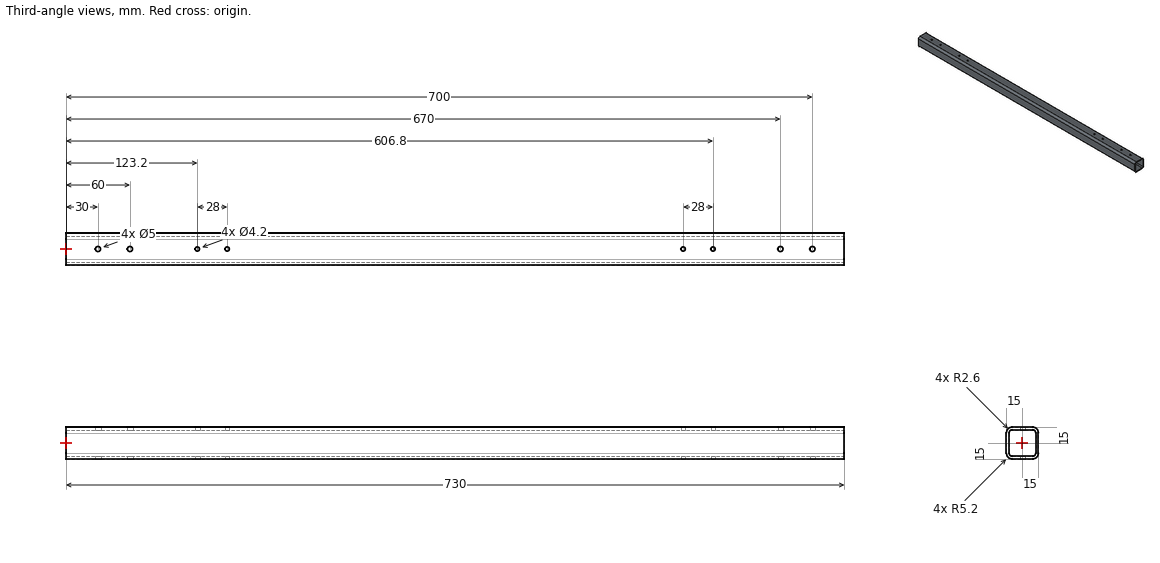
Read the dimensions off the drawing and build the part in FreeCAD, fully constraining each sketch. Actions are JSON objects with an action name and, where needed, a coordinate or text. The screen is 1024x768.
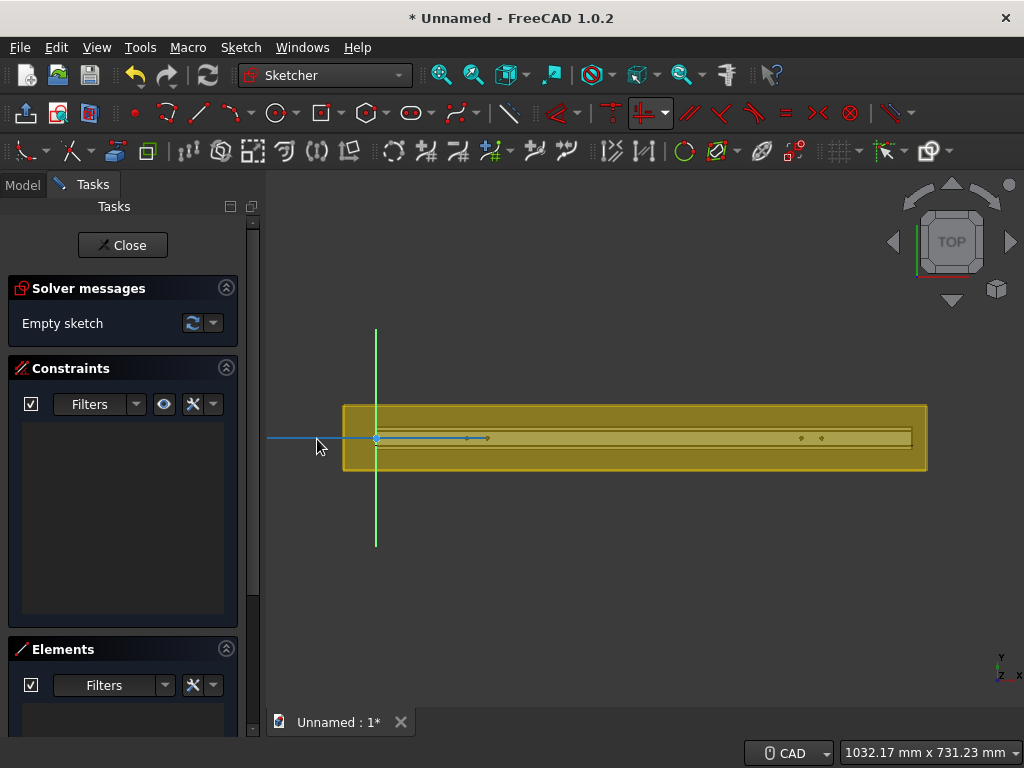
{"action": "left_click", "coordinate": [276, 114]}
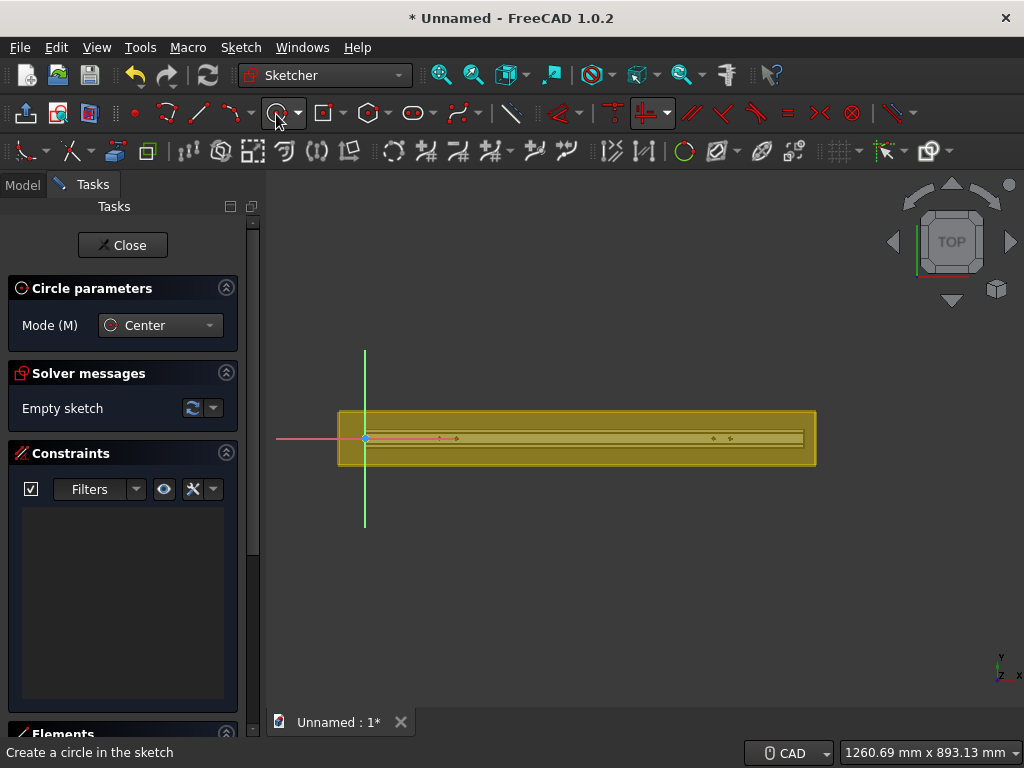
{"action": "scroll", "coordinate": [383, 439], "scroll_direction": "up", "scroll_amount": 14}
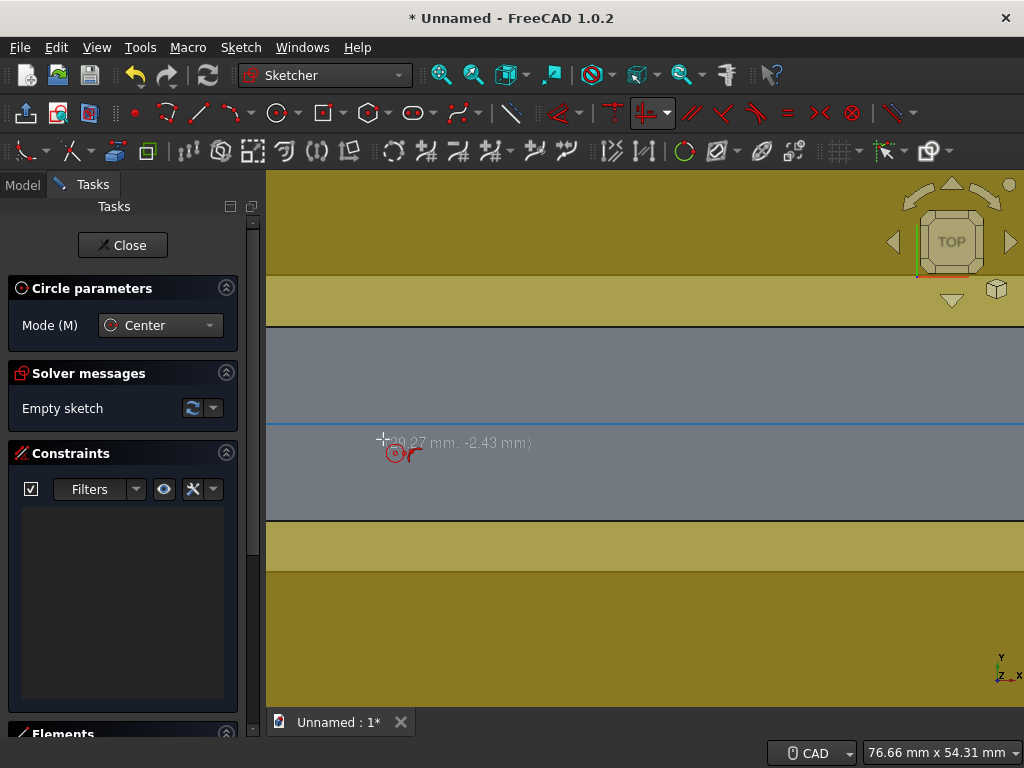
{"action": "scroll", "coordinate": [383, 439], "scroll_direction": "down", "scroll_amount": 14}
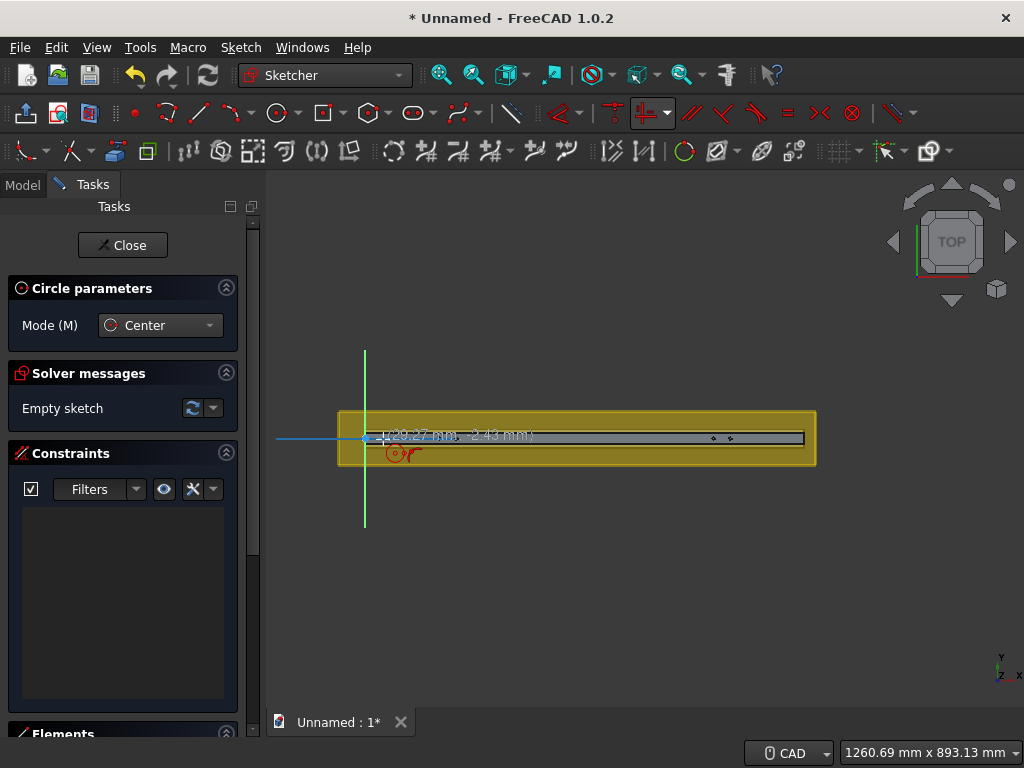
{"action": "left_click", "coordinate": [383, 439]}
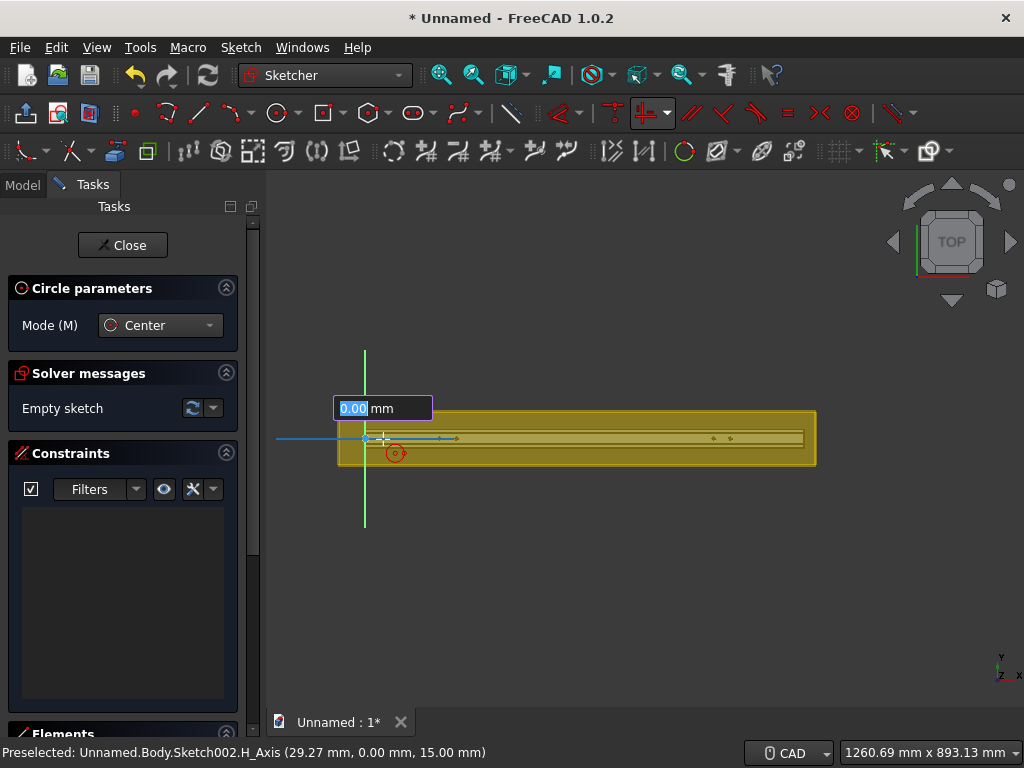
{"action": "scroll", "coordinate": [383, 440], "scroll_direction": "up", "scroll_amount": 13}
{"action": "mouse_move", "coordinate": [380, 433]}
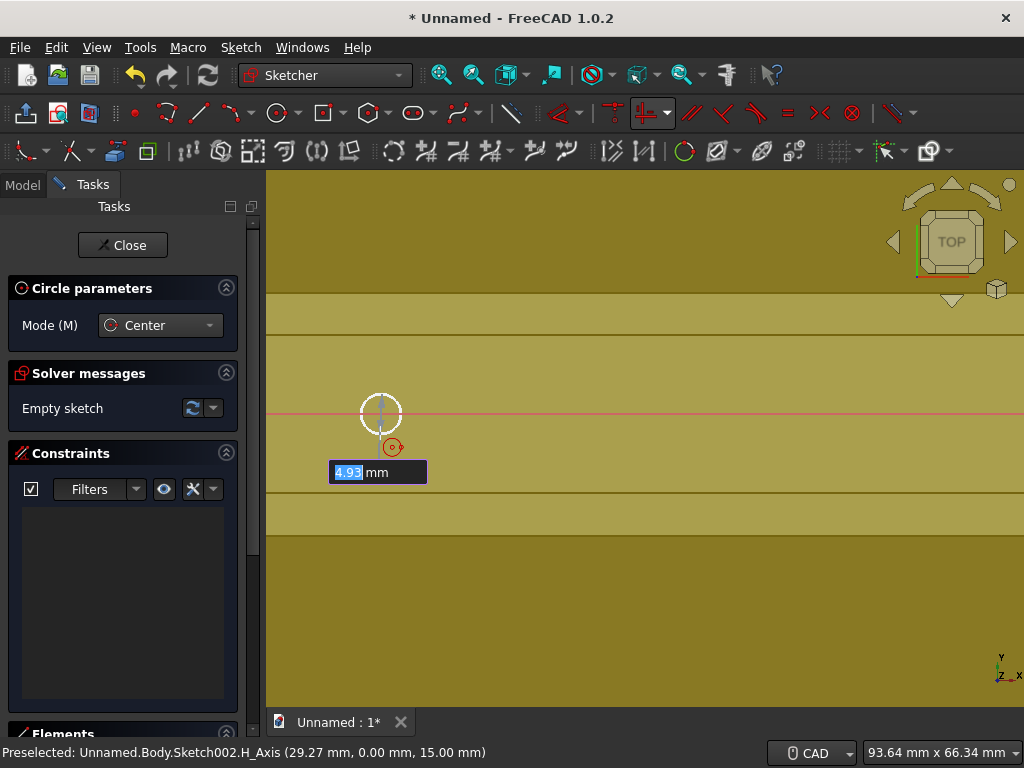
{"action": "type", "text": "5"}
{"action": "key", "text": "Return"}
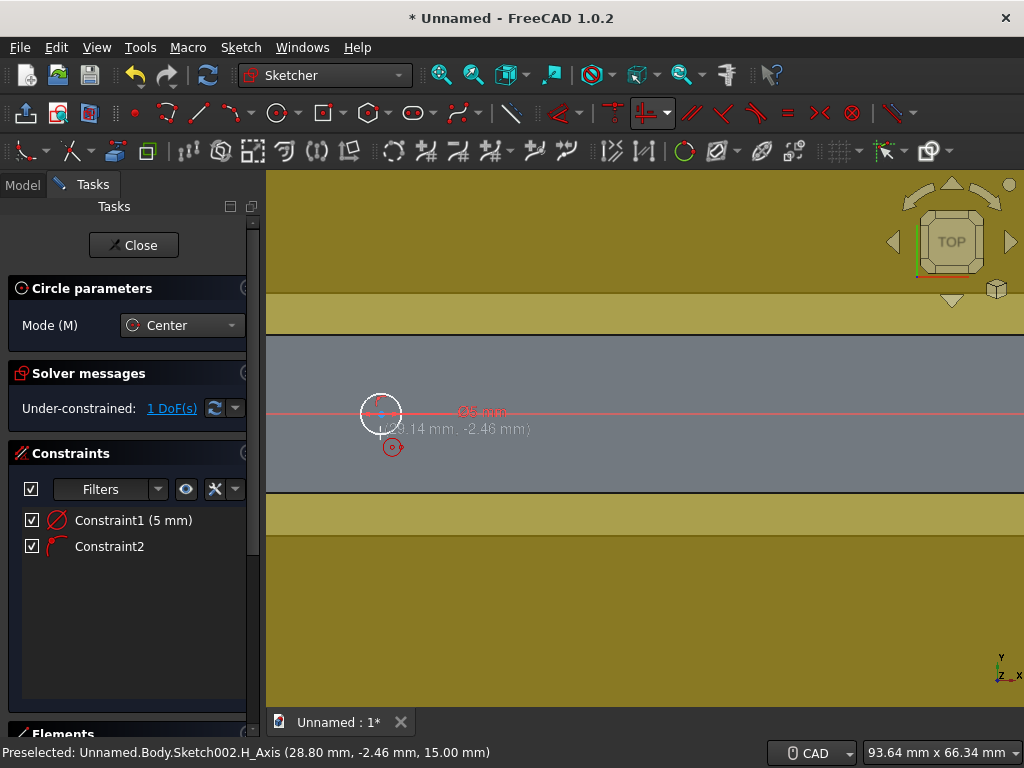
{"action": "scroll", "coordinate": [383, 440], "scroll_direction": "down", "scroll_amount": 13}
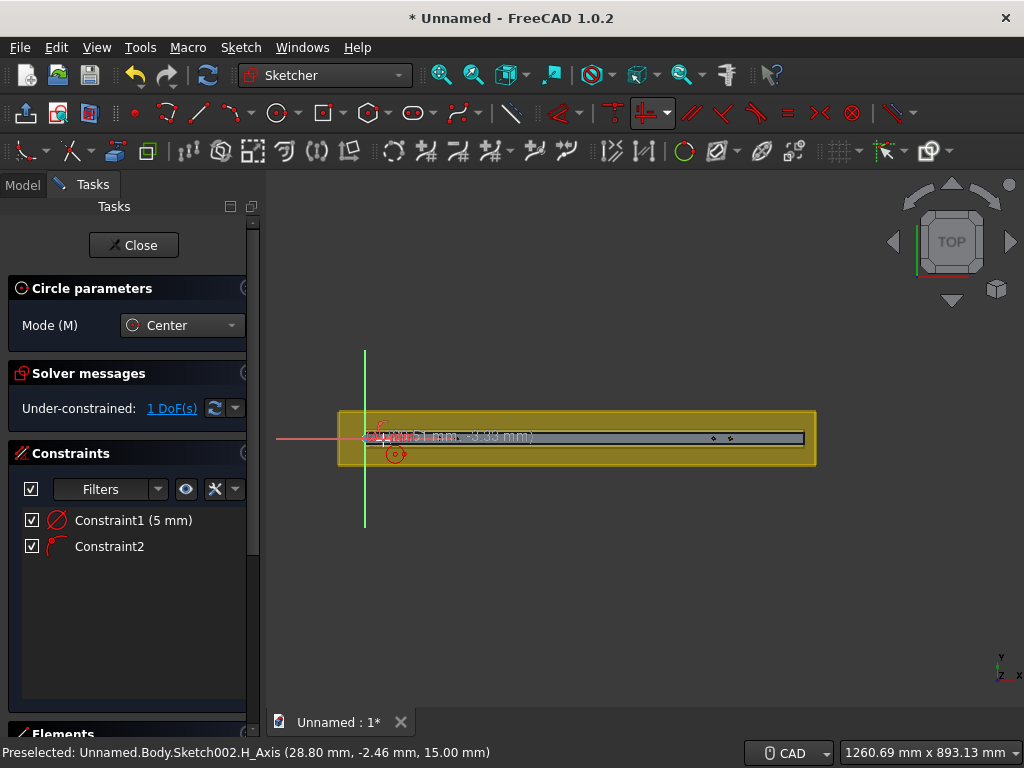
{"action": "left_click", "coordinate": [401, 439]}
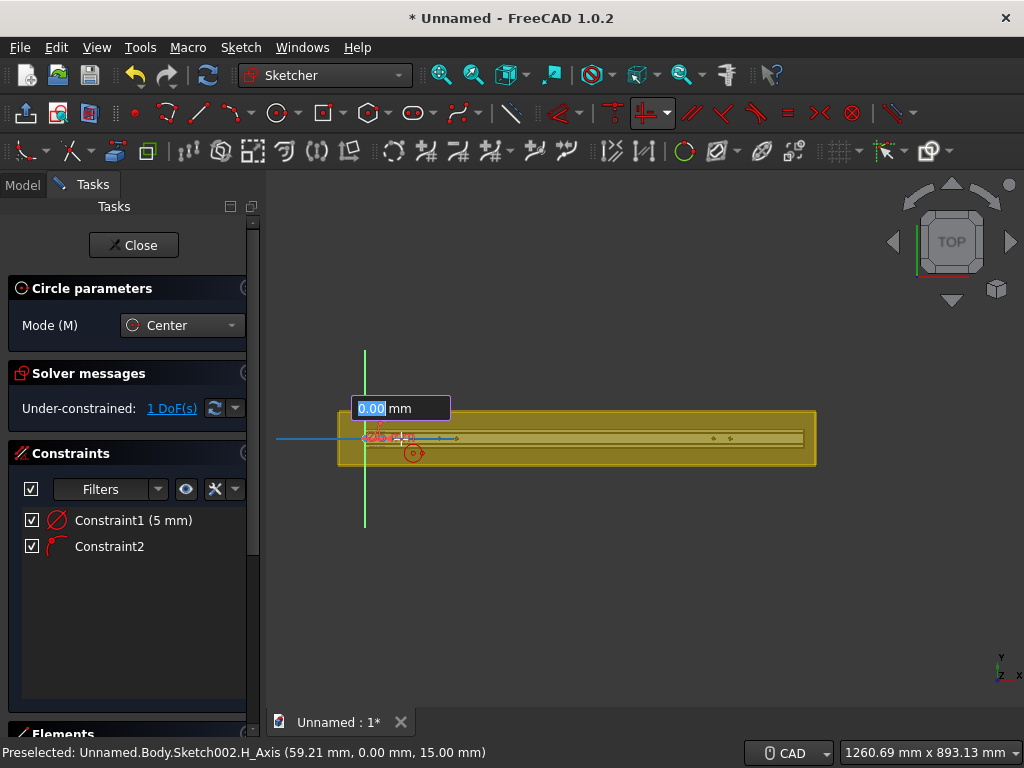
{"action": "scroll", "coordinate": [401, 440], "scroll_direction": "up", "scroll_amount": 13}
{"action": "mouse_move", "coordinate": [398, 433]}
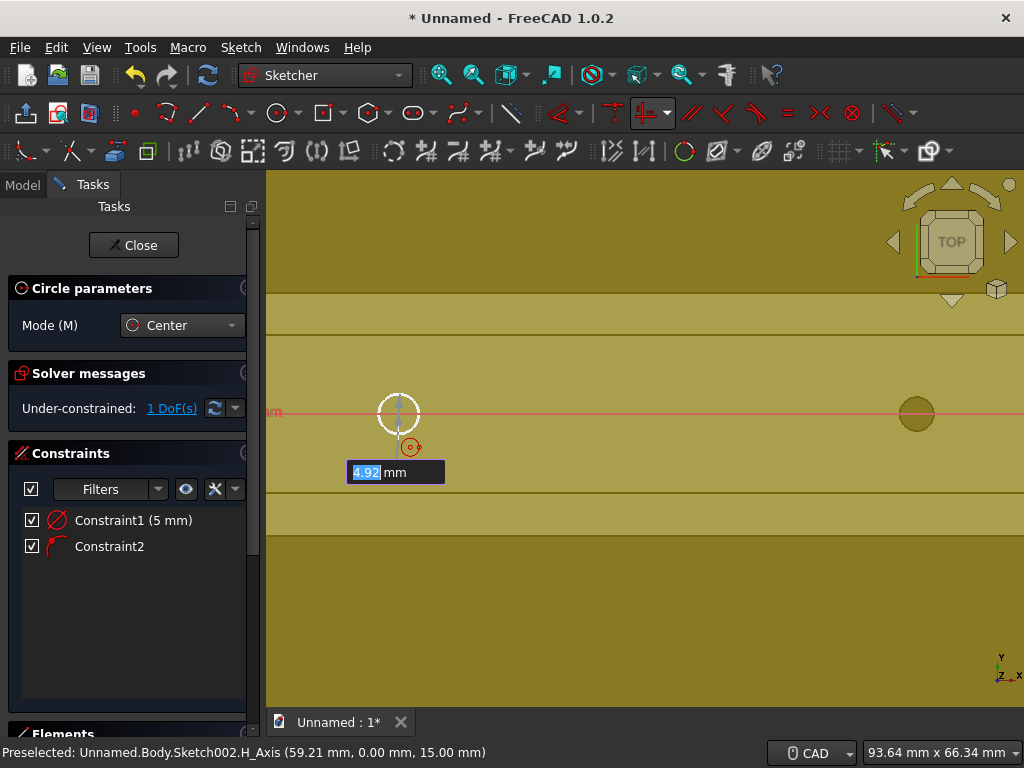
{"action": "type", "text": "5"}
{"action": "key", "text": "Return"}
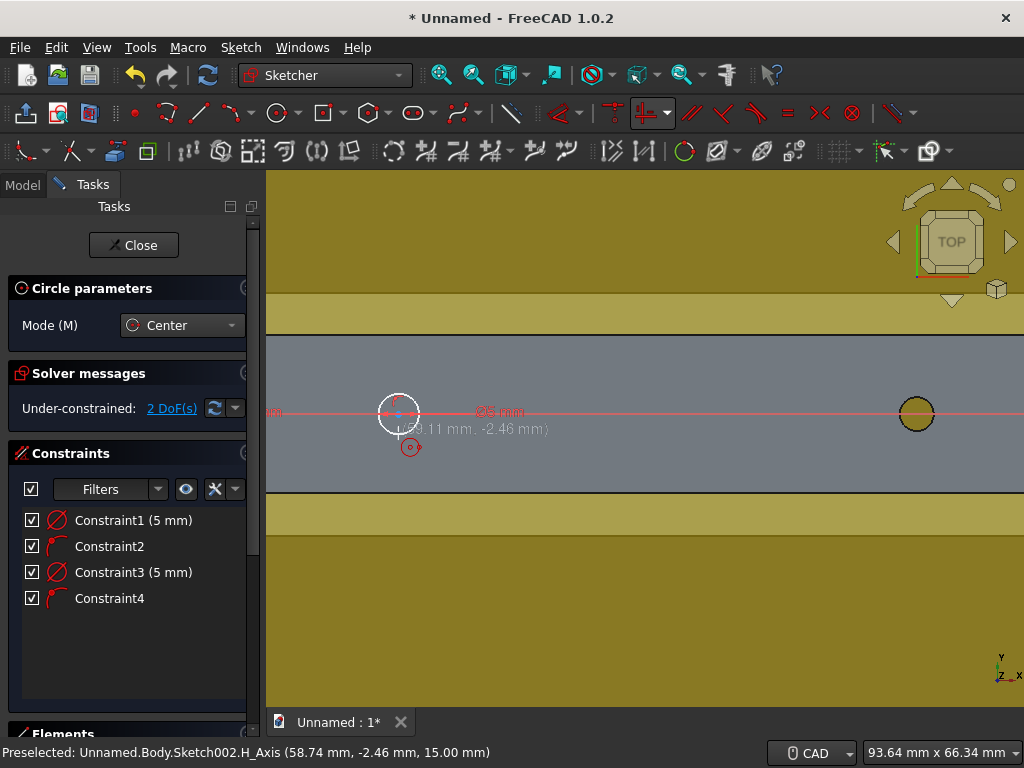
{"action": "scroll", "coordinate": [401, 440], "scroll_direction": "down", "scroll_amount": 13}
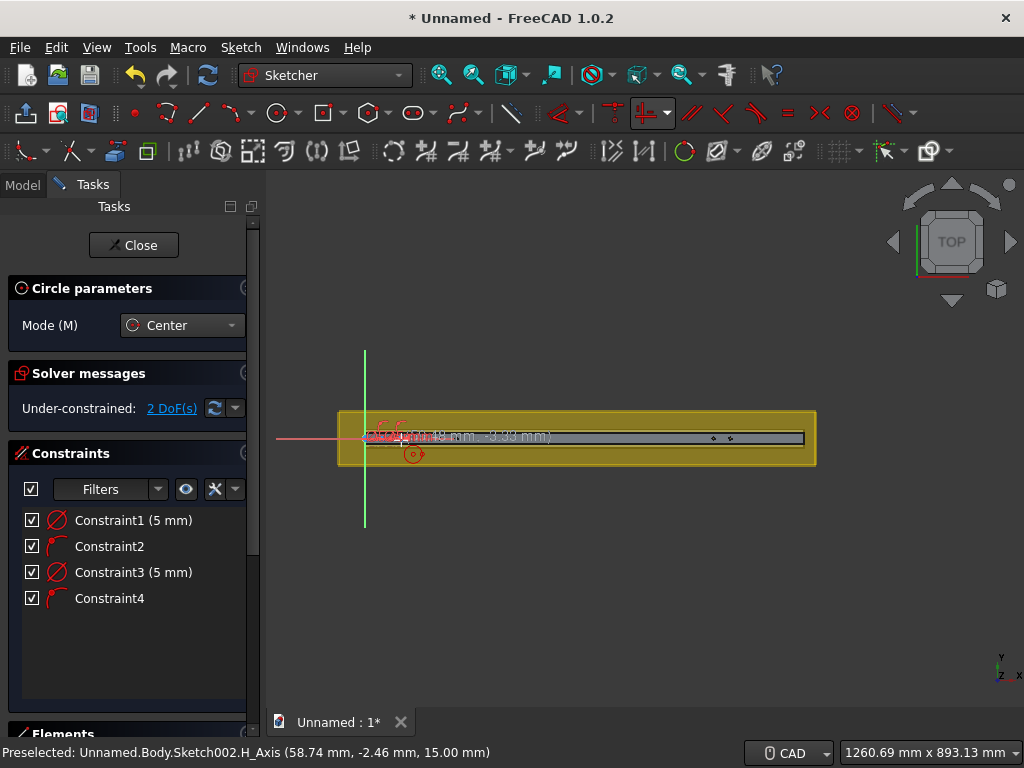
{"action": "scroll", "coordinate": [786, 439], "scroll_direction": "up", "scroll_amount": 14}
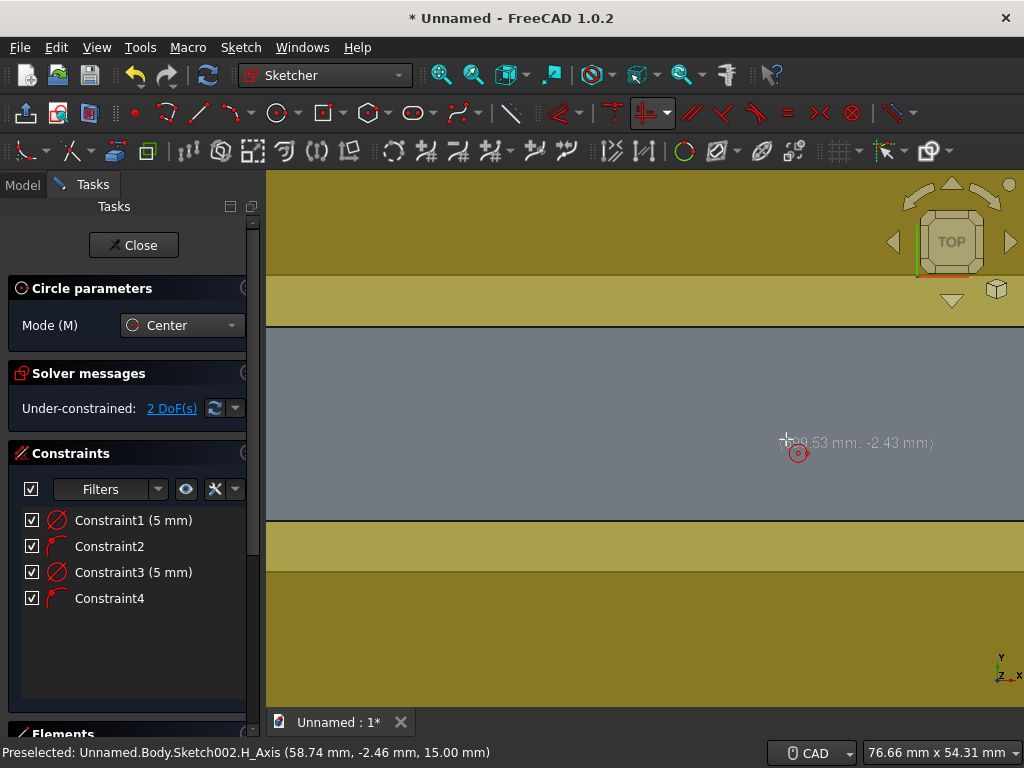
{"action": "scroll", "coordinate": [787, 439], "scroll_direction": "down", "scroll_amount": 14}